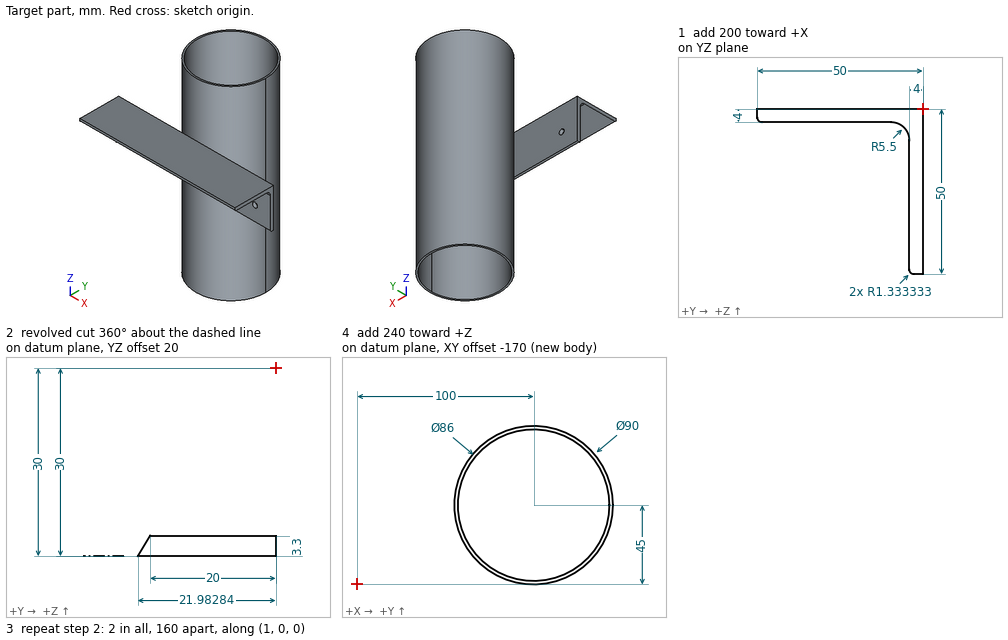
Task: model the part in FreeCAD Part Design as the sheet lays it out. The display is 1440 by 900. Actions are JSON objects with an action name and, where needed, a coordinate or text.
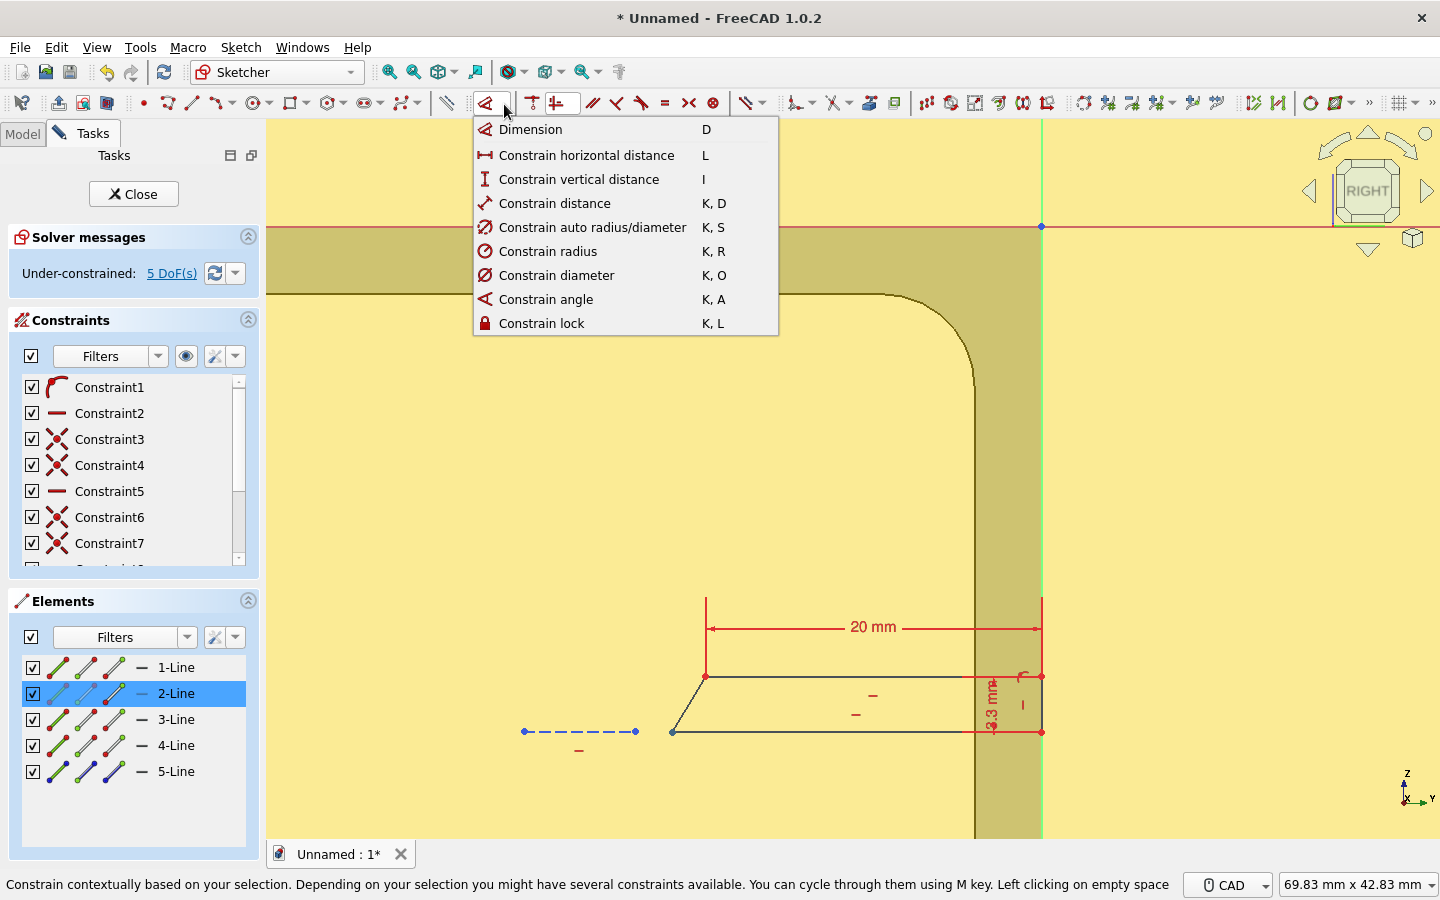
{"action": "left_click", "coordinate": [626, 179]}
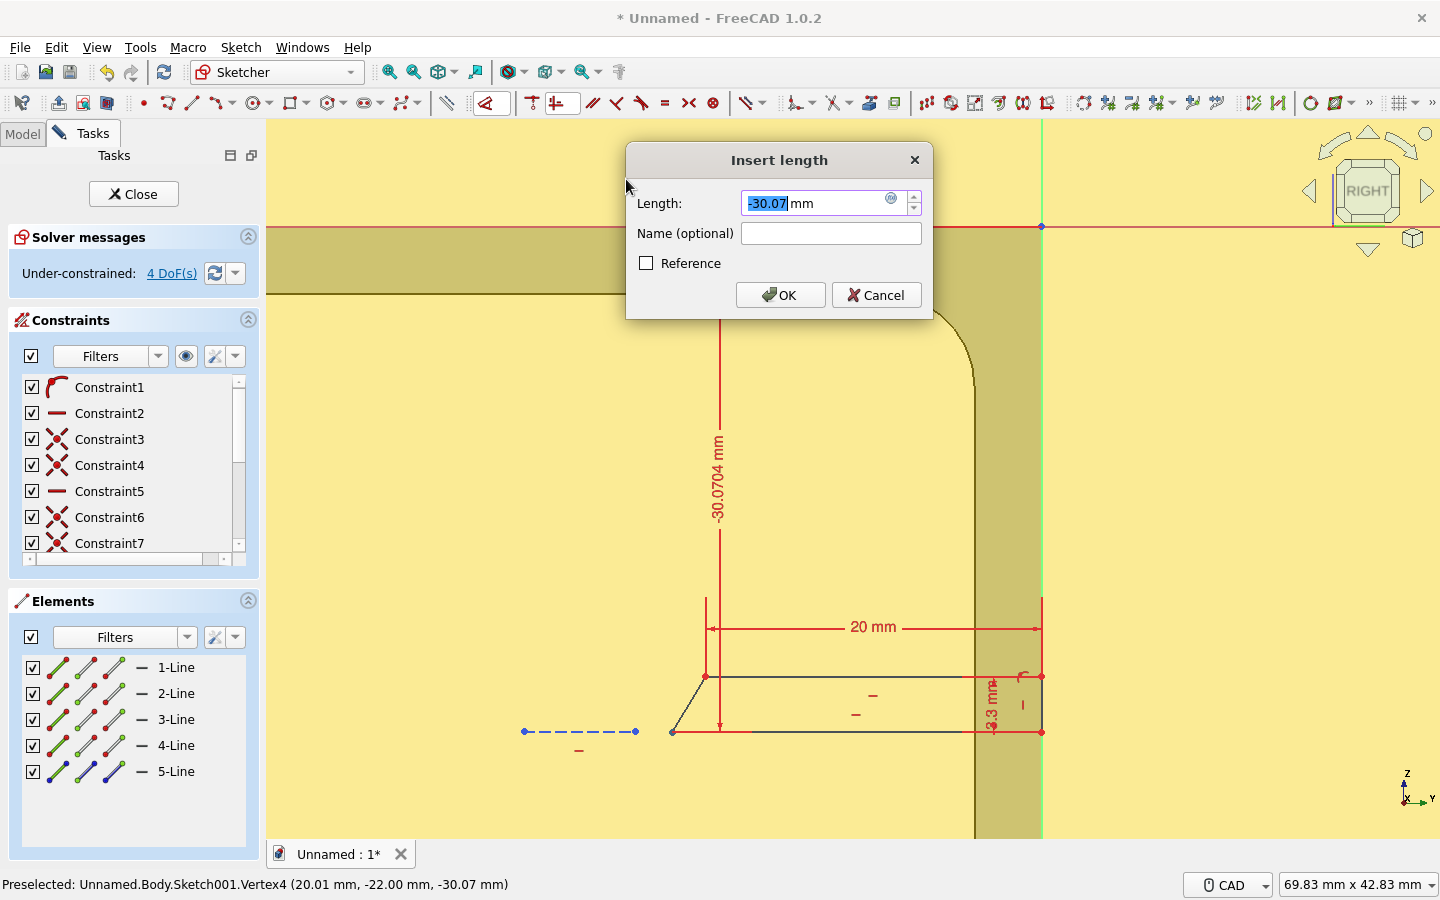
{"action": "type", "text": "-30"}
{"action": "key", "text": "Return"}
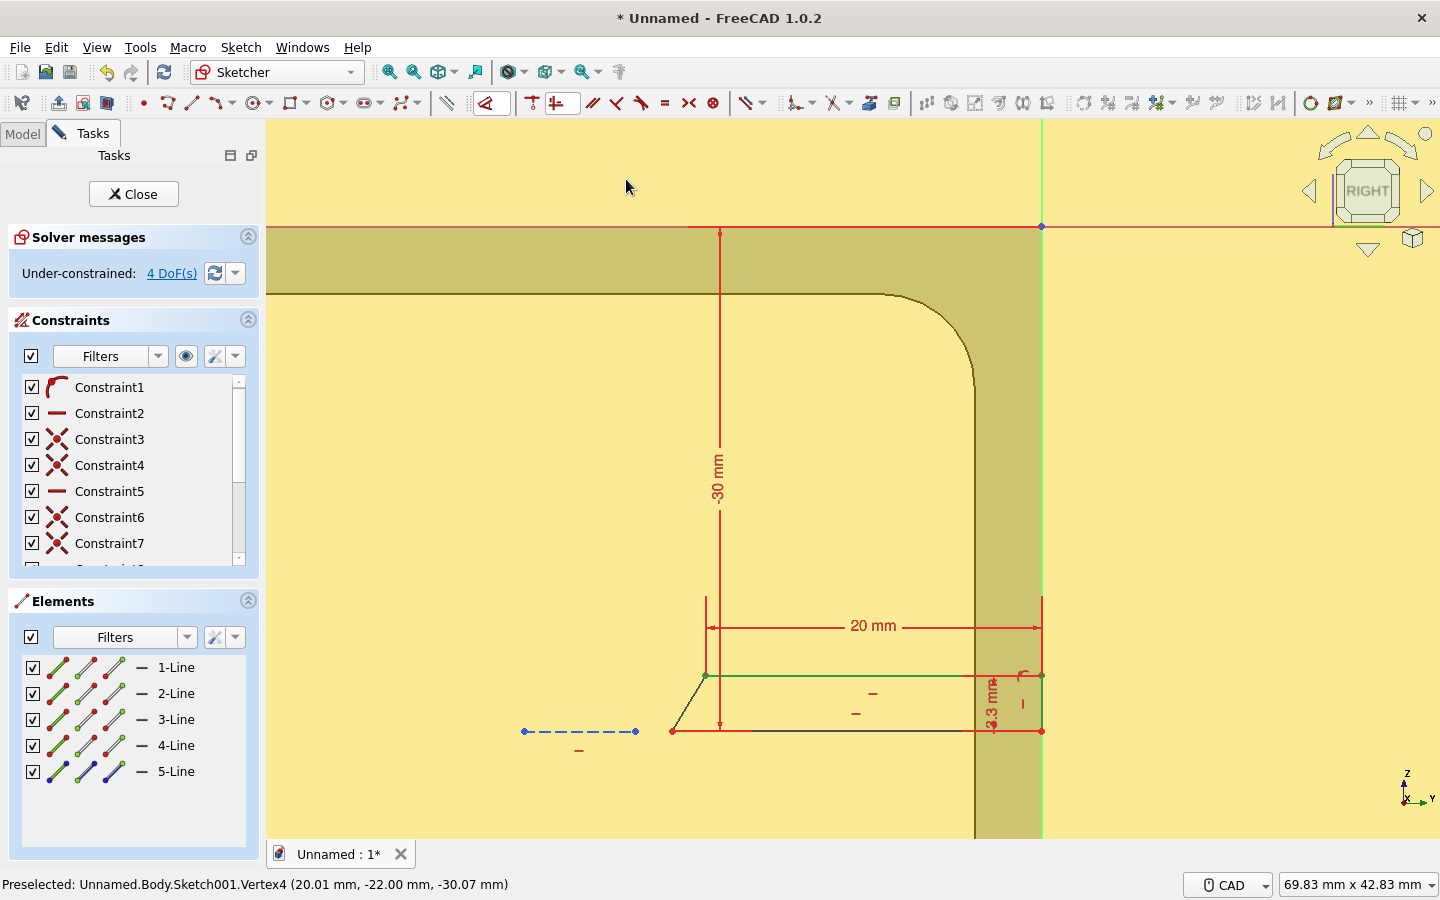
{"action": "left_click", "coordinate": [635, 732]}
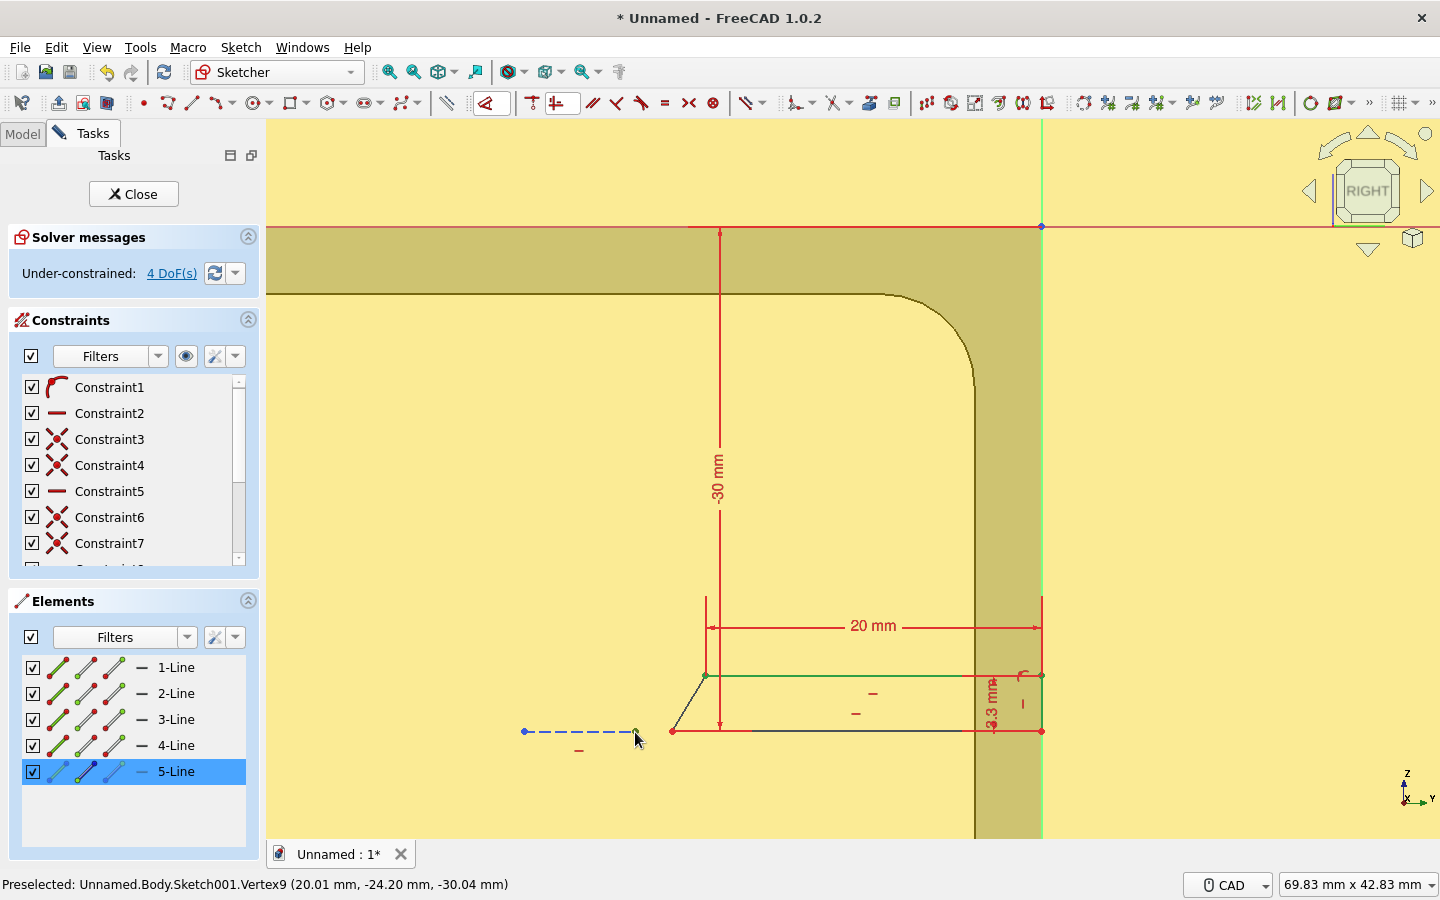
{"action": "key", "text": "i"}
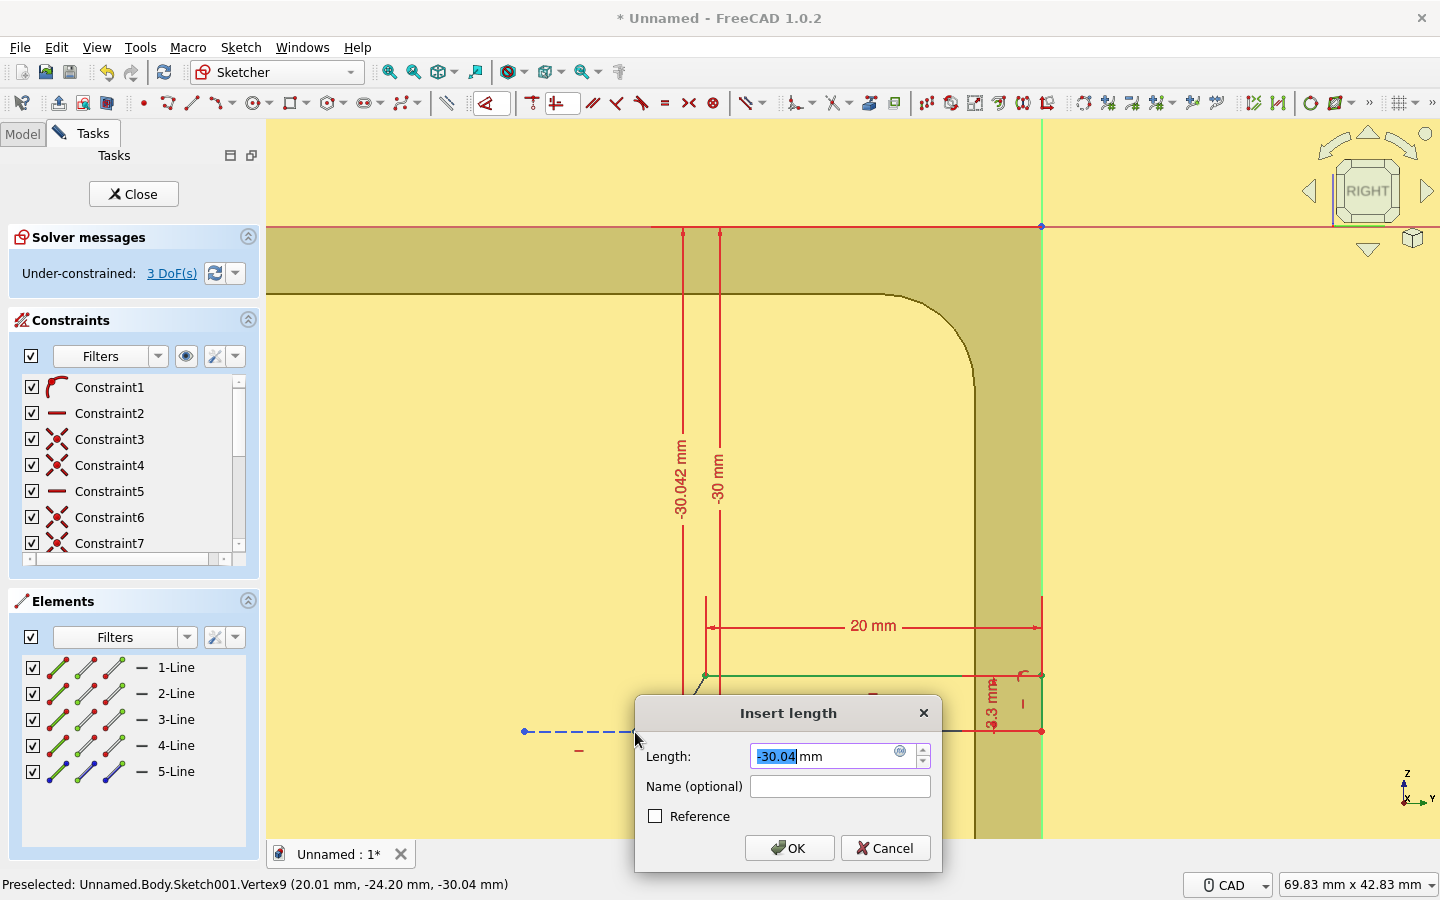
{"action": "type", "text": "-30"}
{"action": "key", "text": "Return"}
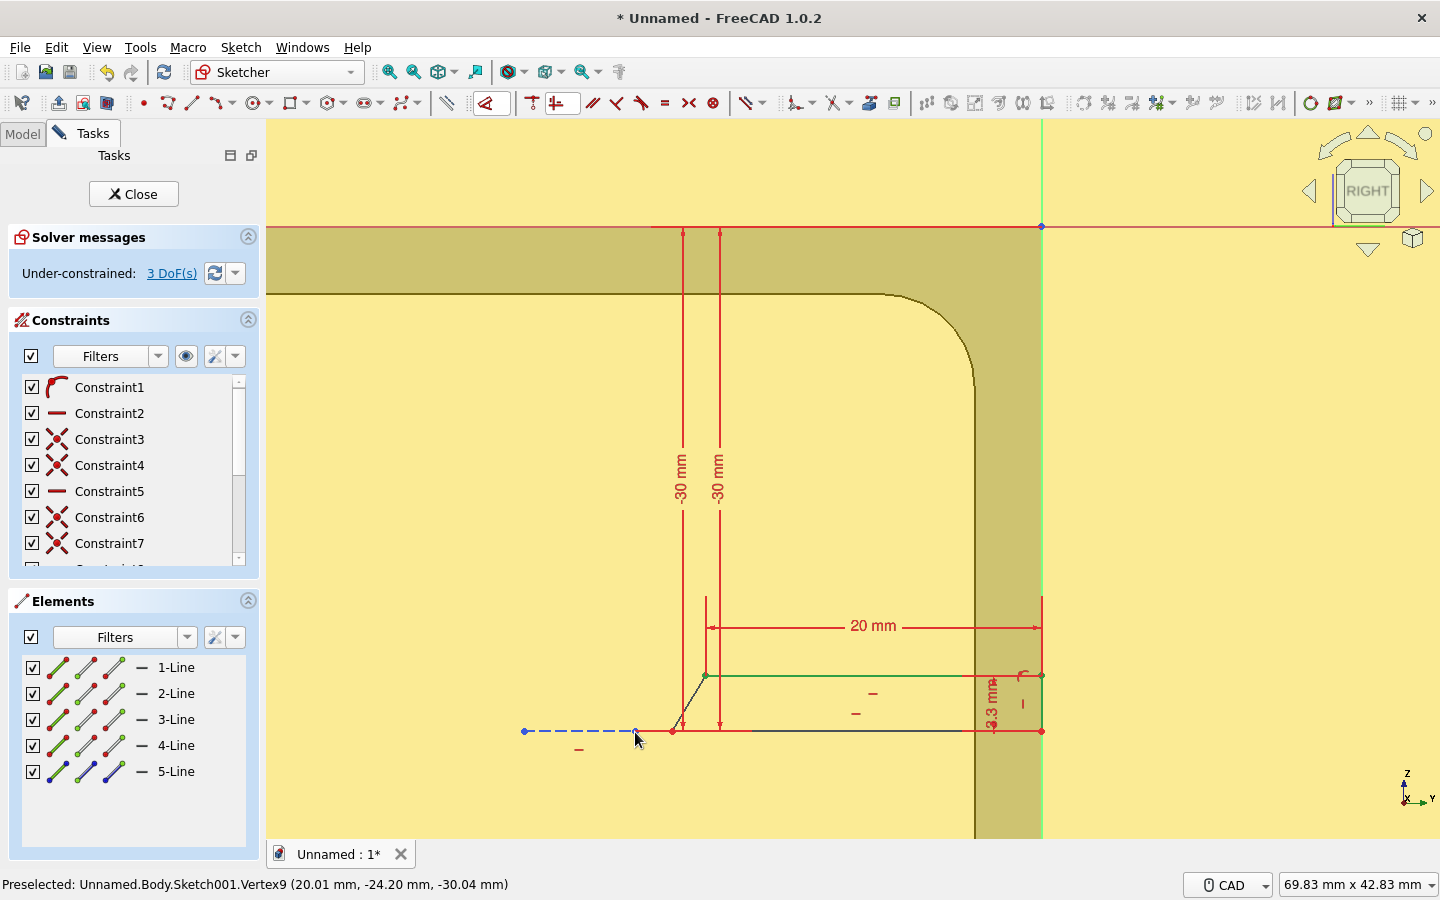
{"action": "left_click", "coordinate": [783, 731]}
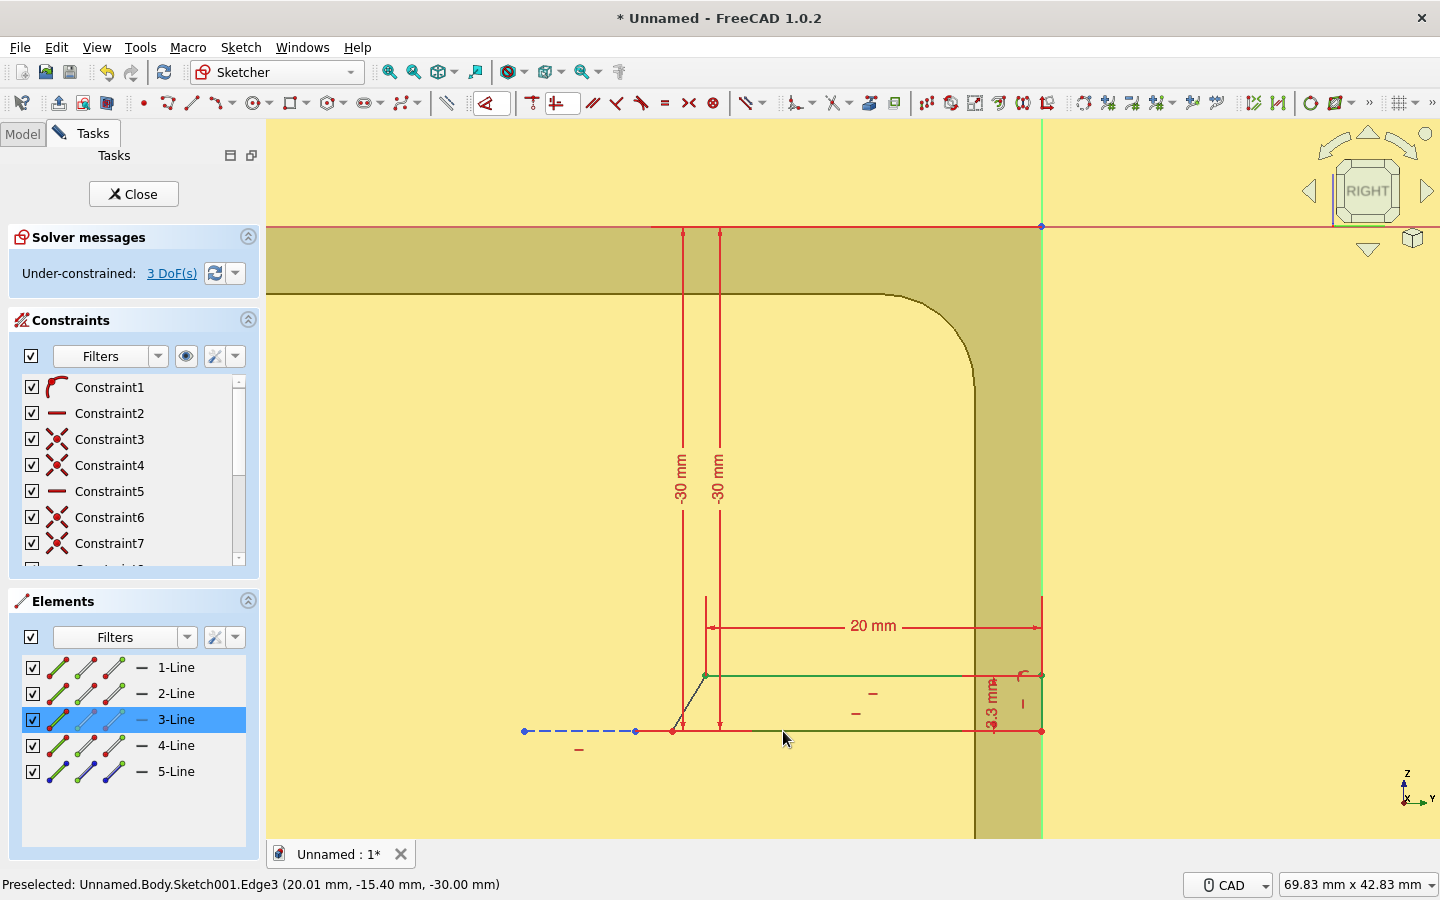
{"action": "left_click", "coordinate": [504, 104]}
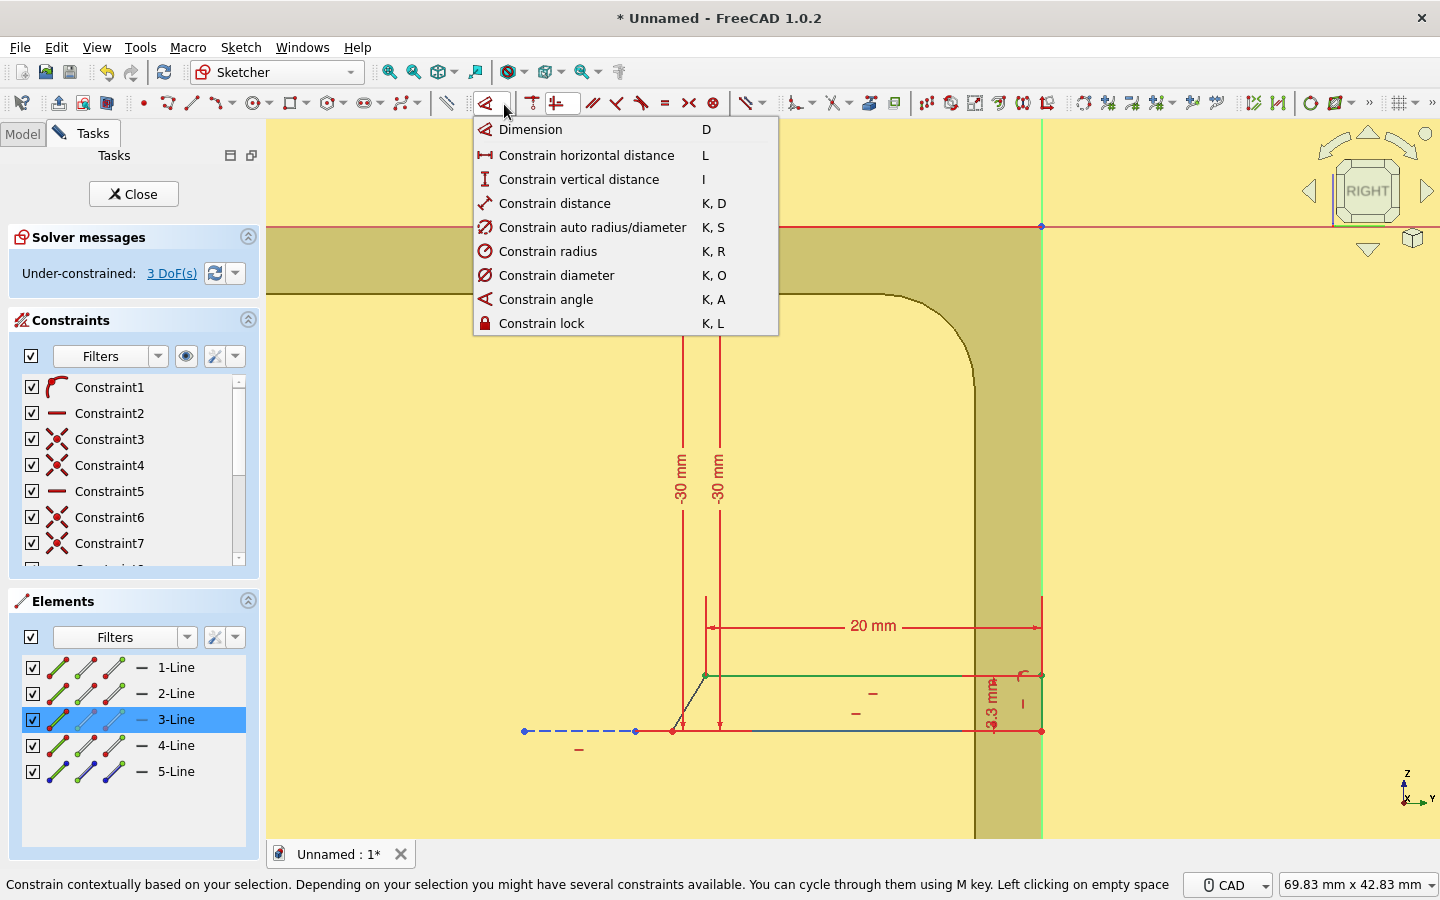
{"action": "left_click", "coordinate": [626, 155]}